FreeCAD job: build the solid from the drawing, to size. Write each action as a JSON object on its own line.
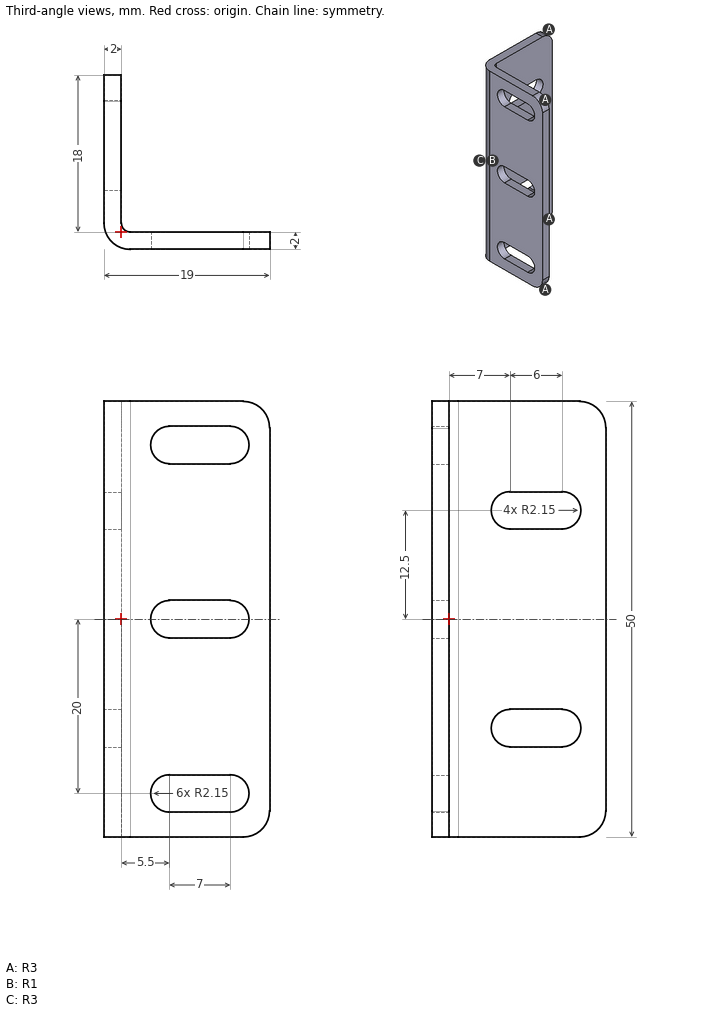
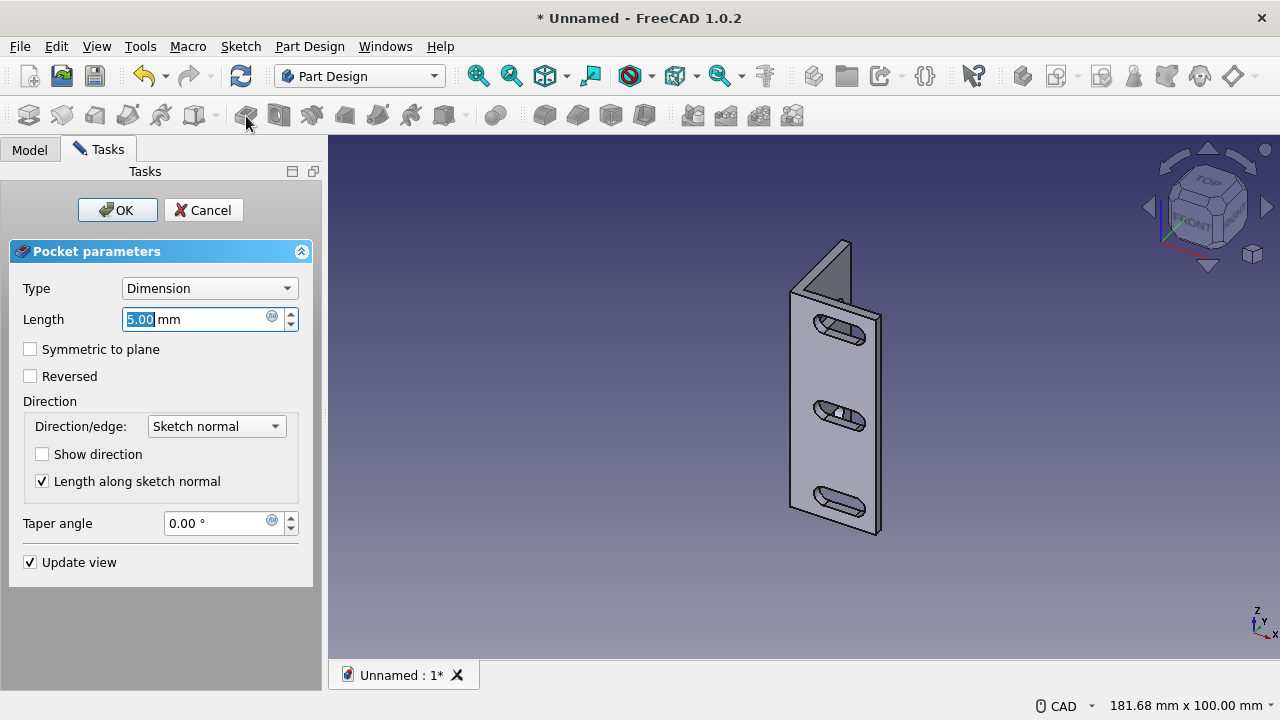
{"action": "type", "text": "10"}
{"action": "key", "text": "Tab"}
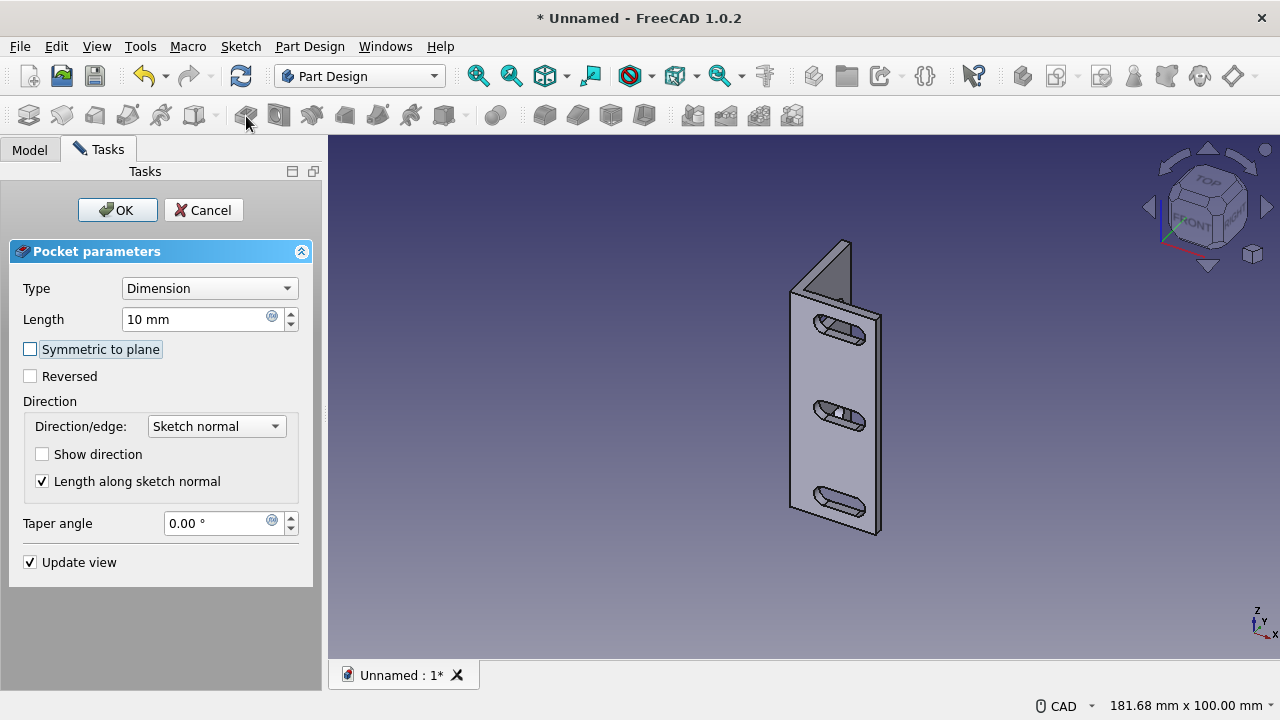
{"action": "left_click", "coordinate": [118, 210]}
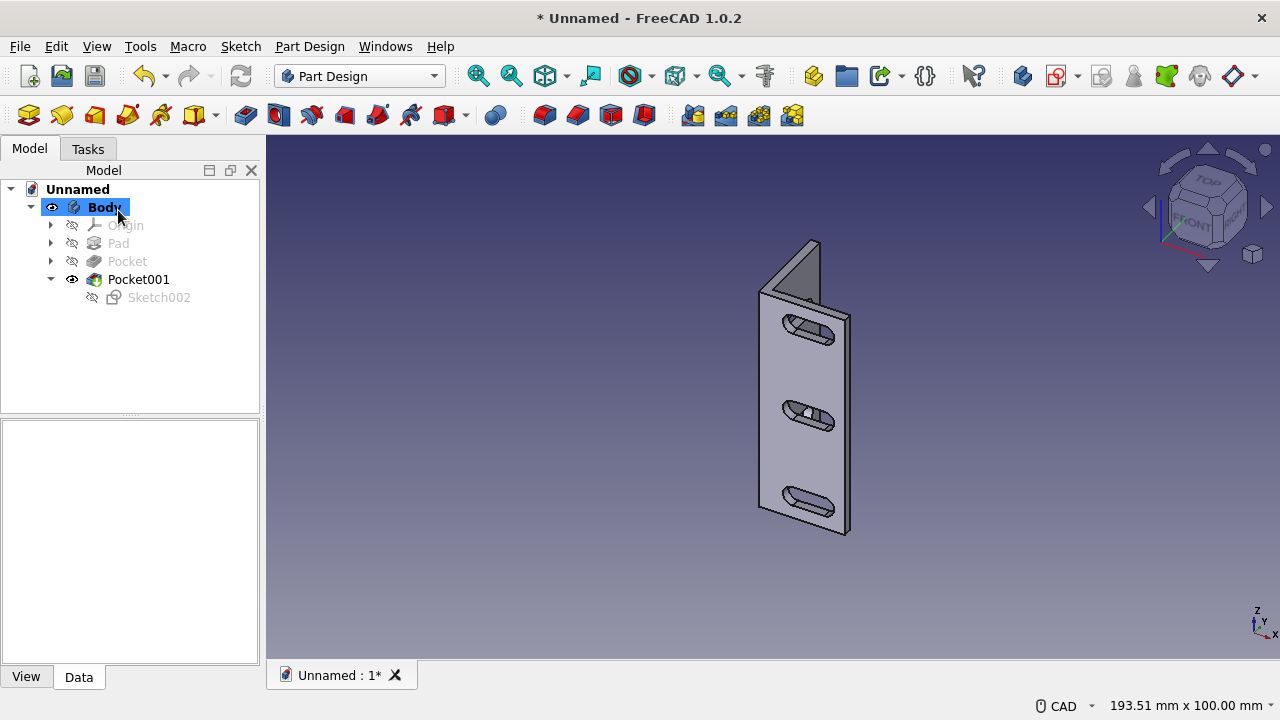
{"action": "scroll", "coordinate": [816, 240], "scroll_direction": "up", "scroll_amount": 7}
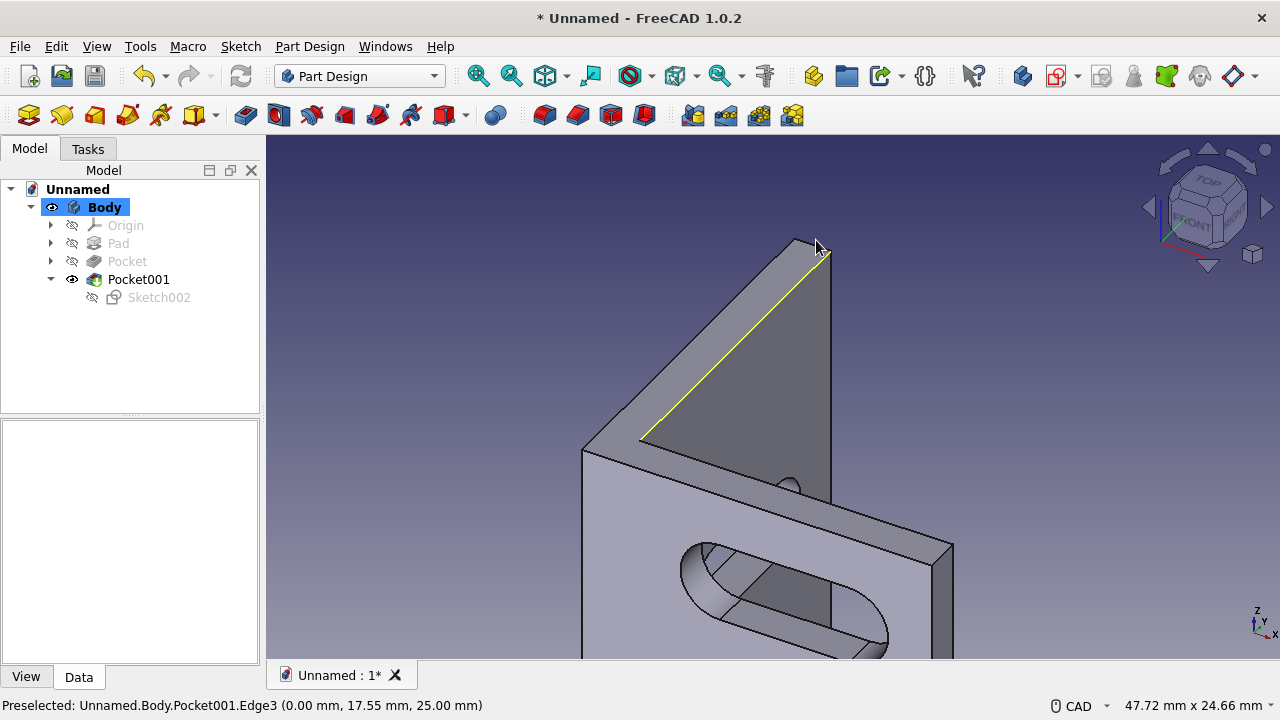
{"action": "left_click", "coordinate": [942, 554]}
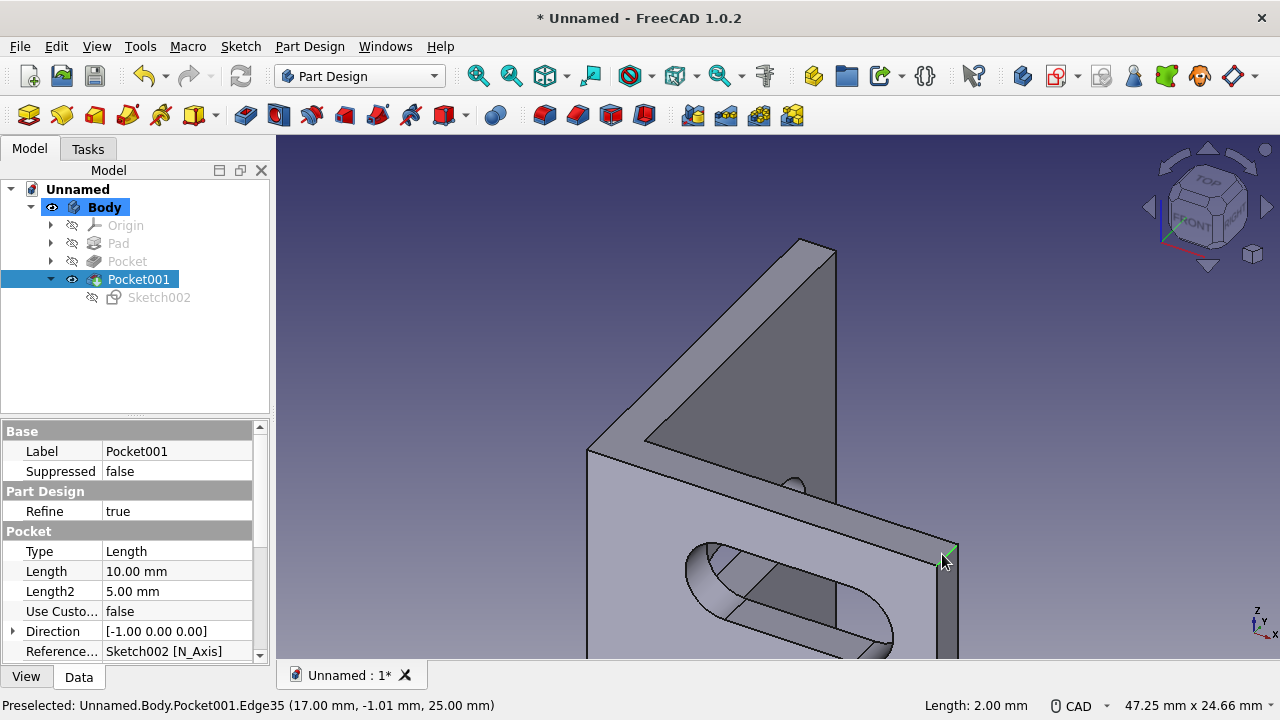
{"action": "left_click", "coordinate": [479, 76]}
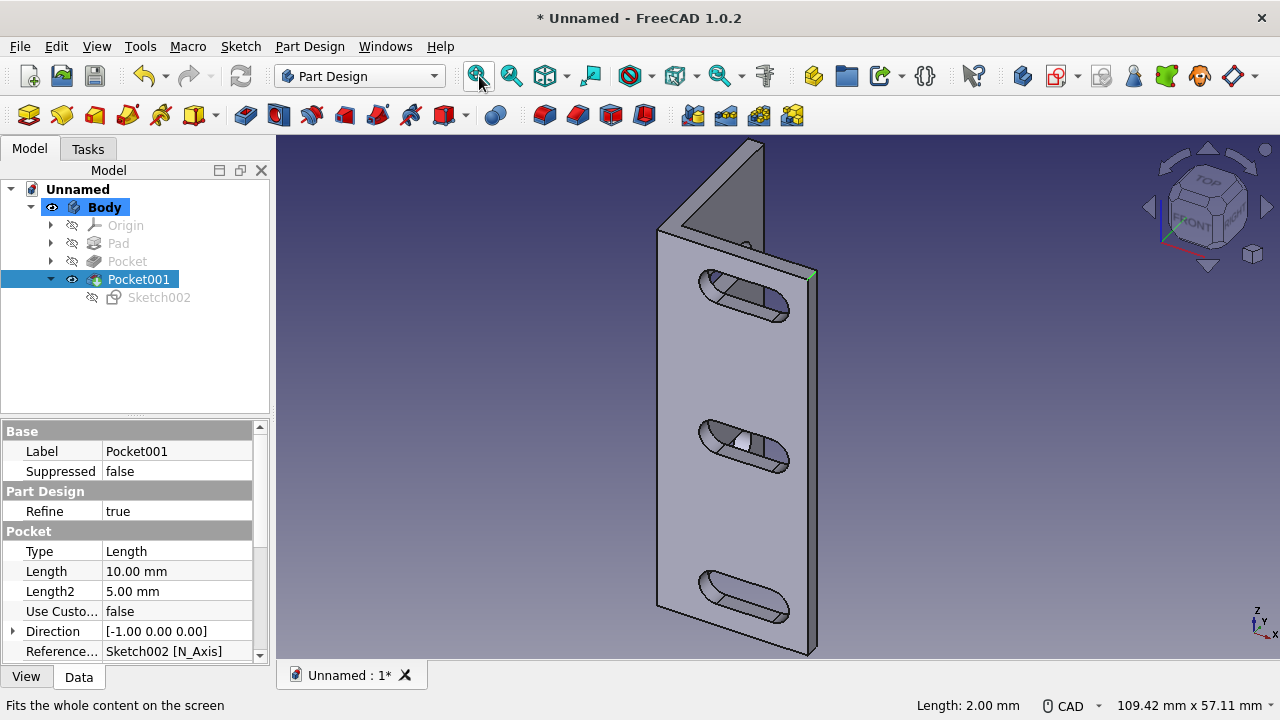
{"action": "key", "text": "0"}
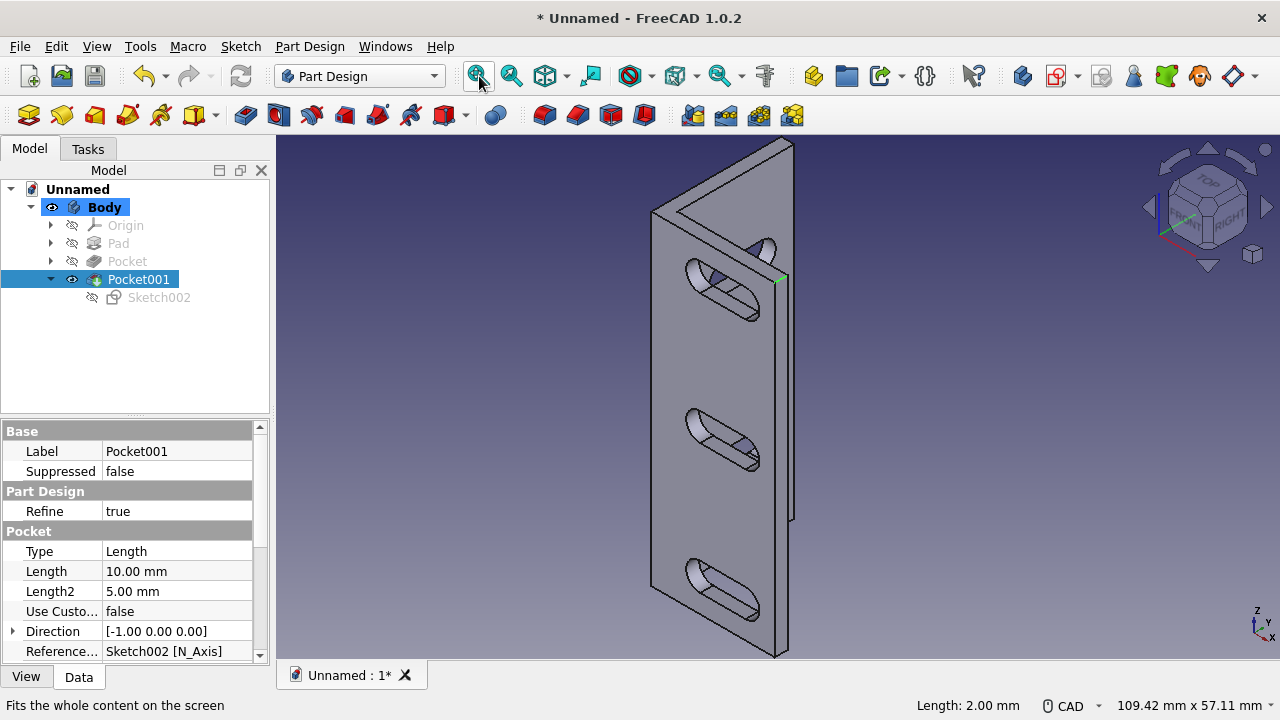
{"action": "key", "text": "2"}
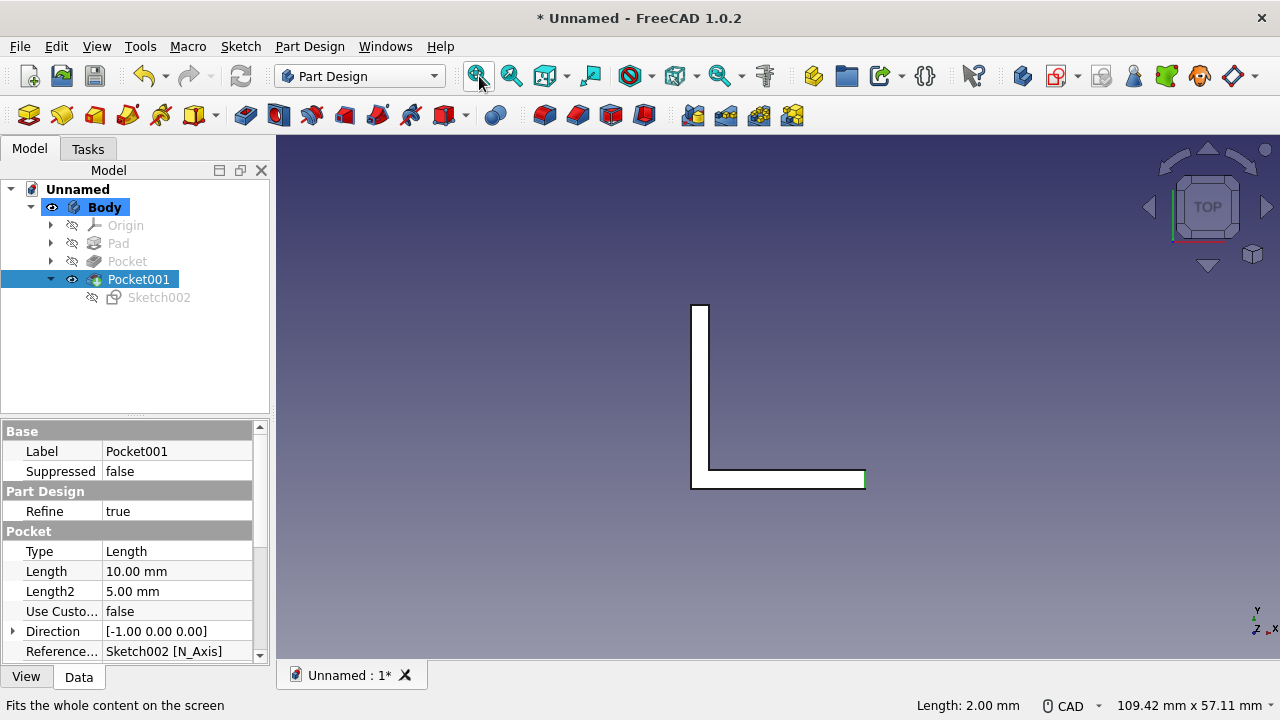
{"action": "left_click", "coordinate": [479, 76]}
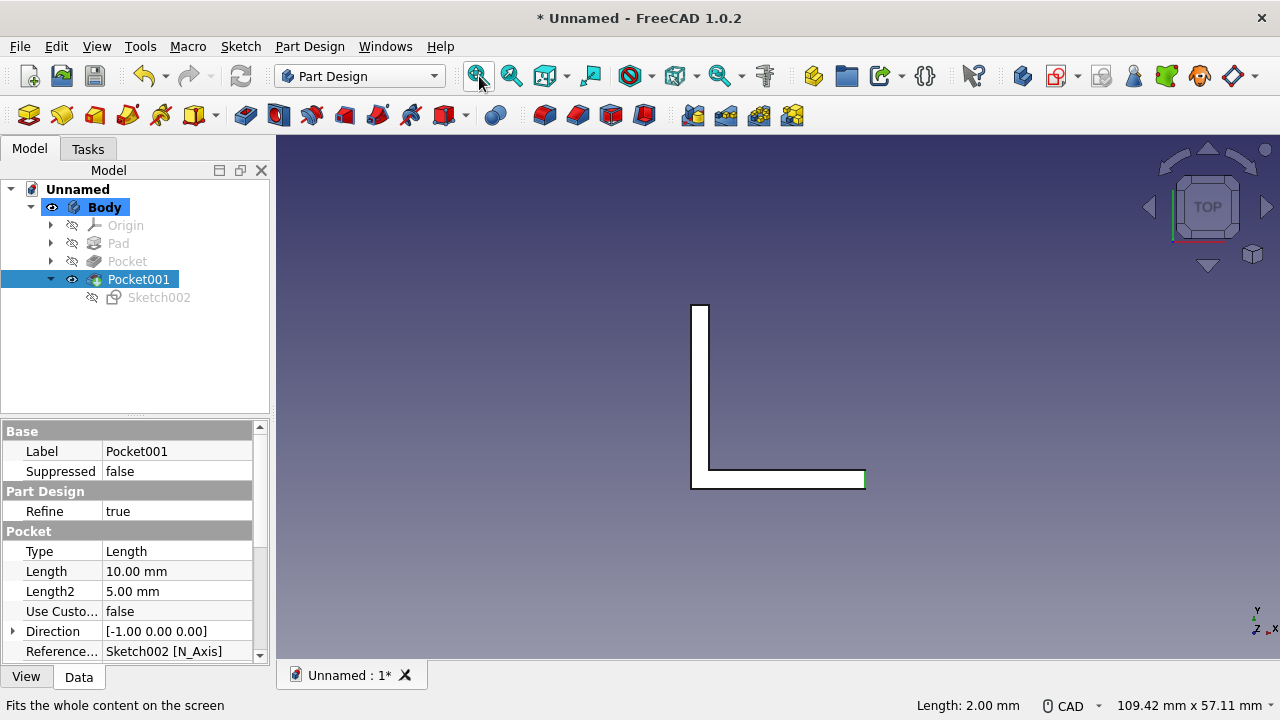
{"action": "left_click", "coordinate": [700, 304], "text": "ctrl"}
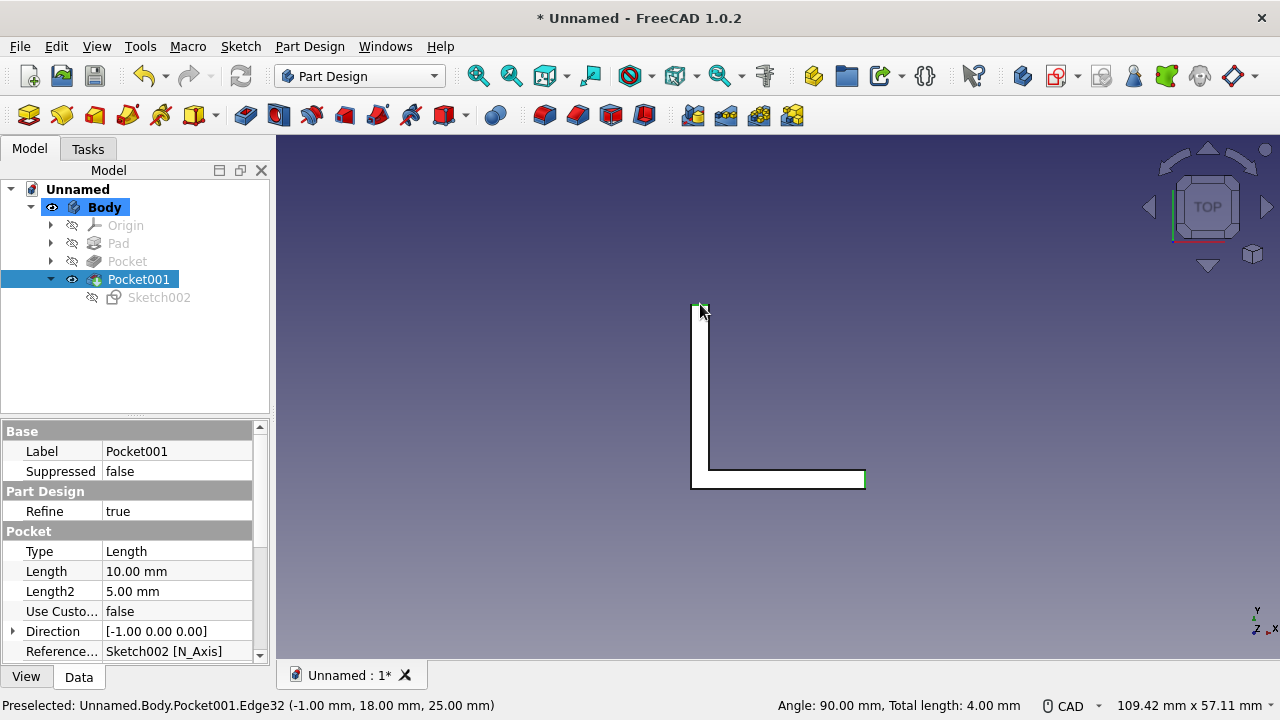
{"action": "scroll", "coordinate": [700, 304], "scroll_direction": "up", "scroll_amount": 4}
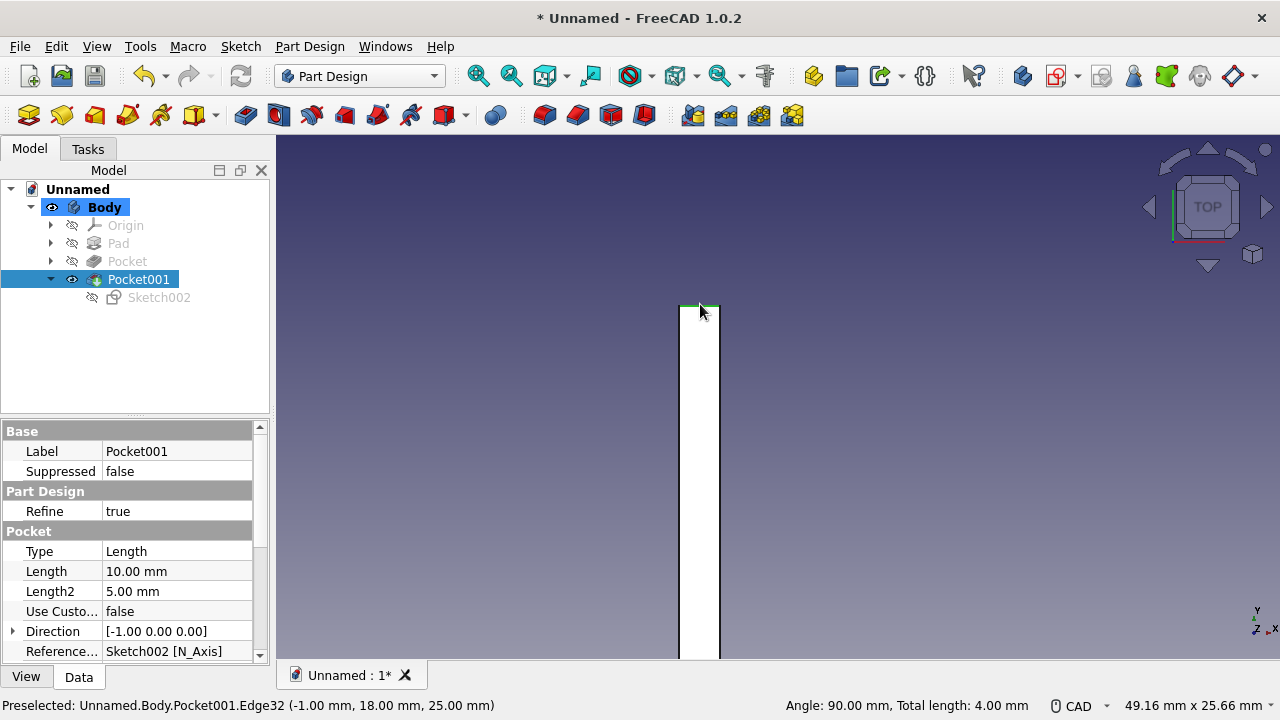
{"action": "left_click", "coordinate": [479, 76]}